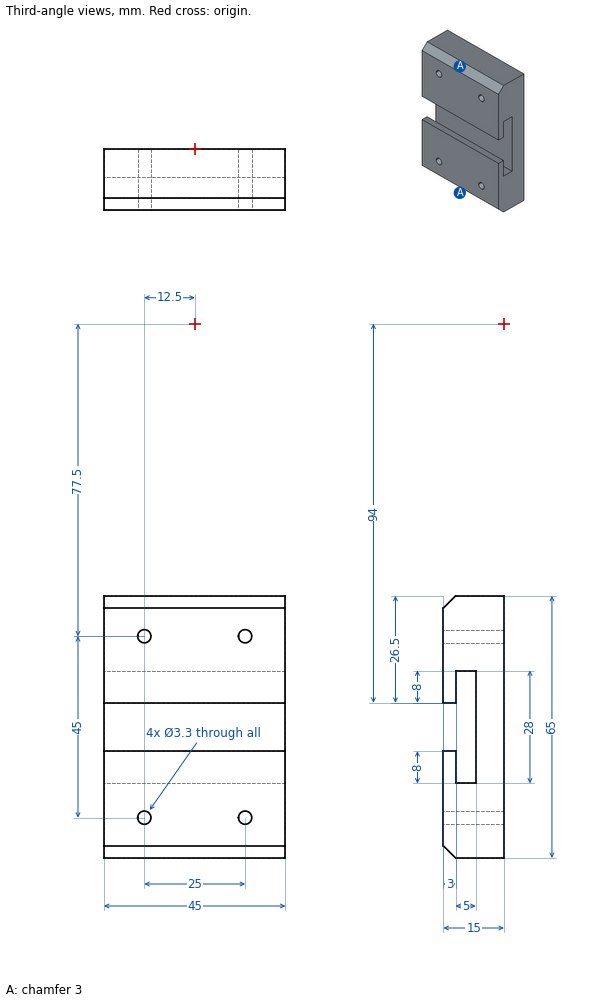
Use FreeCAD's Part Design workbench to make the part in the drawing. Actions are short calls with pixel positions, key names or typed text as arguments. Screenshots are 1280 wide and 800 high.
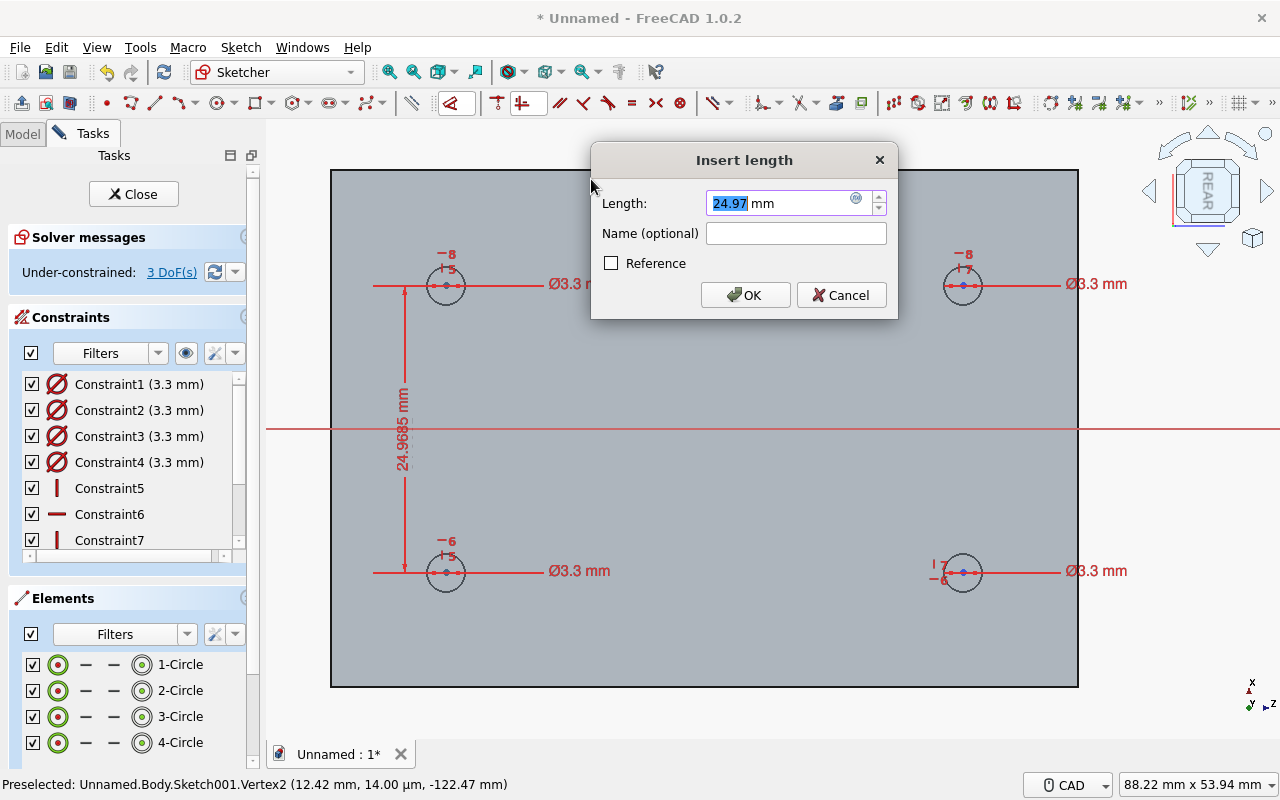
text(25)
key(Return)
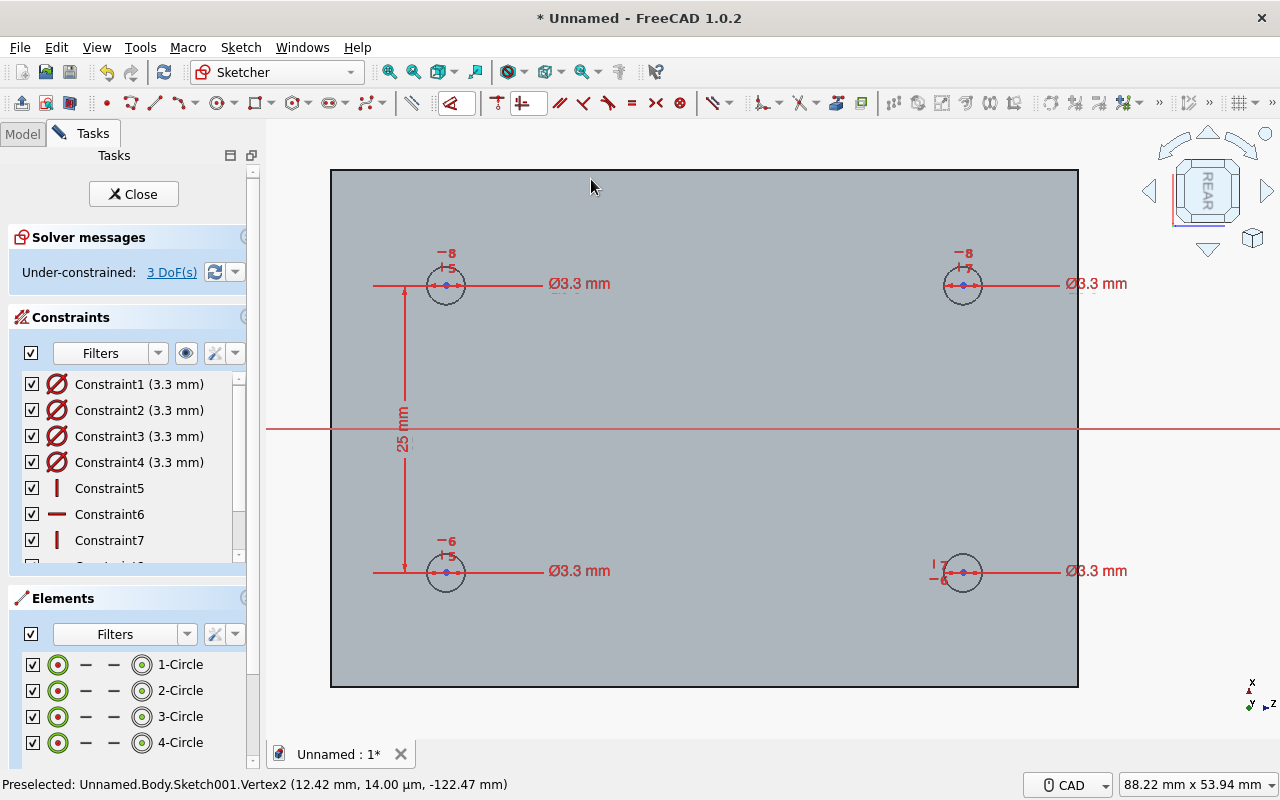
click(446, 573)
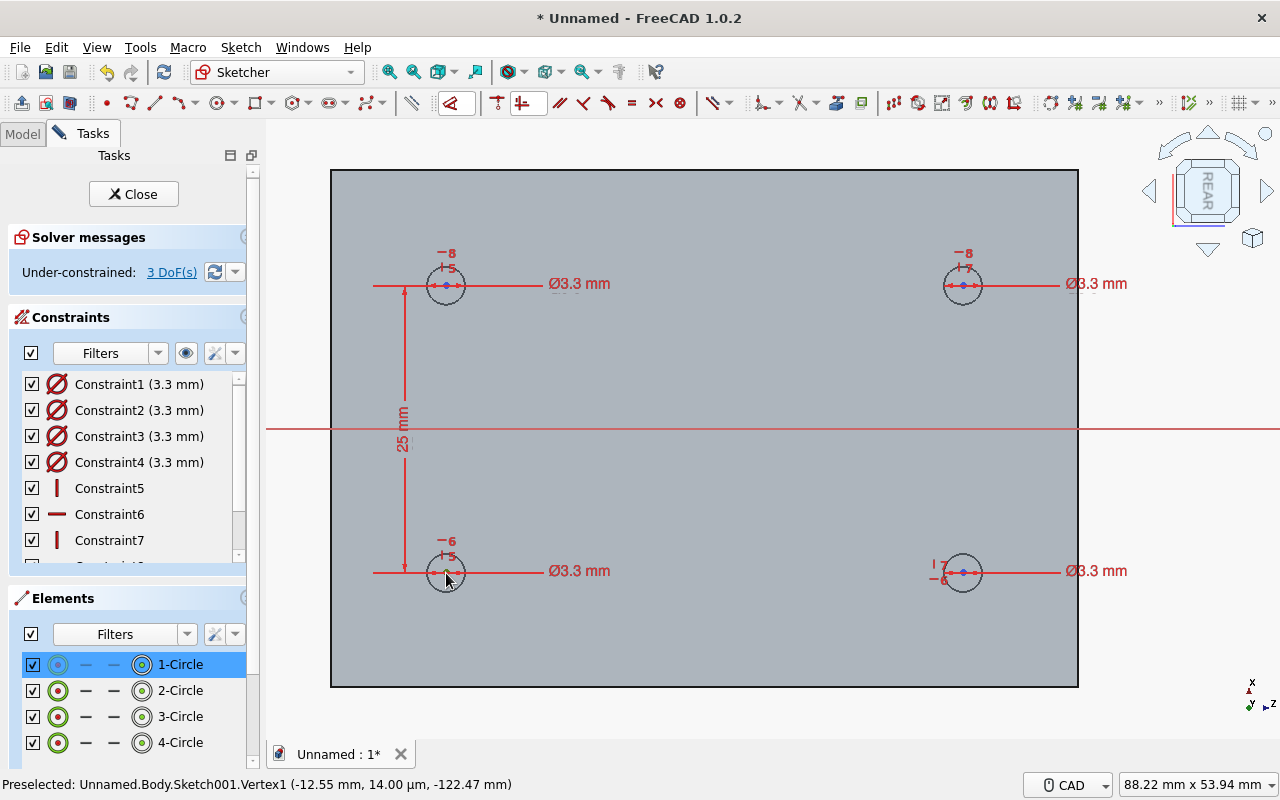
click(963, 573)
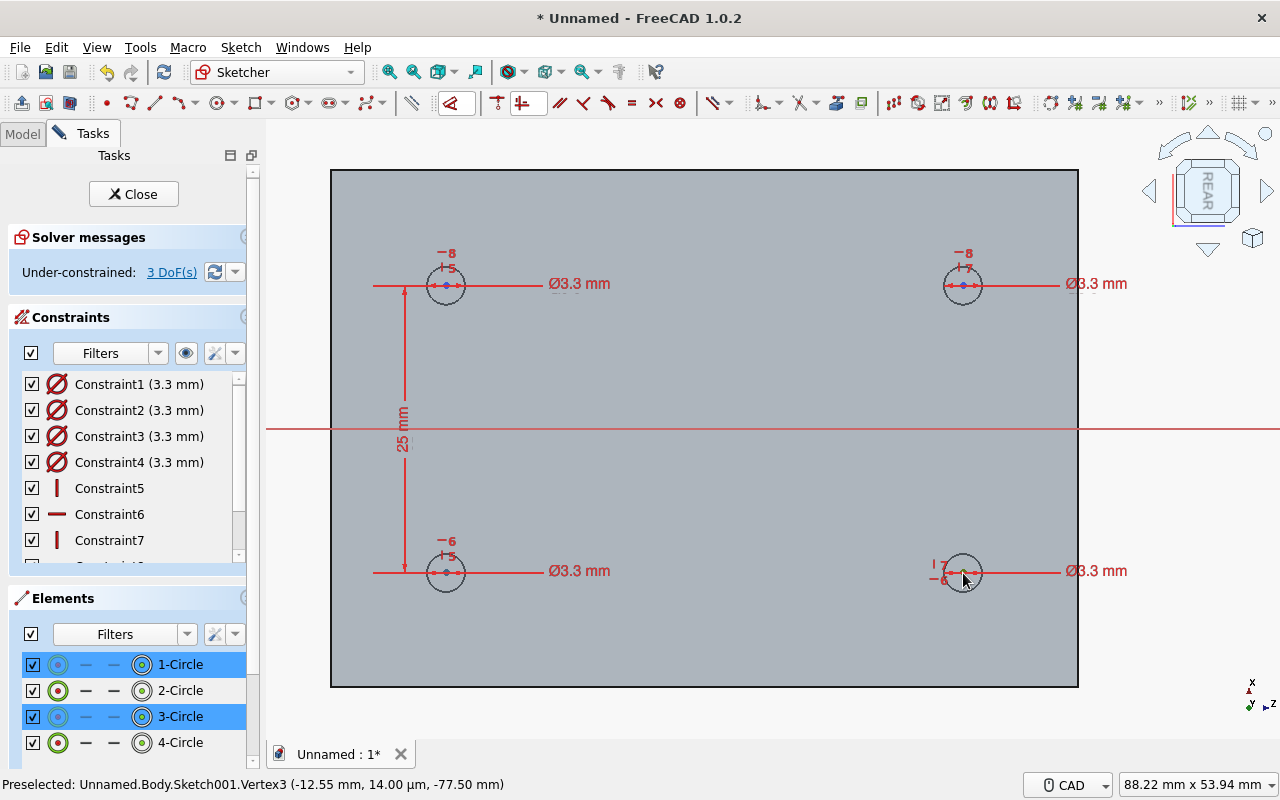
key(l)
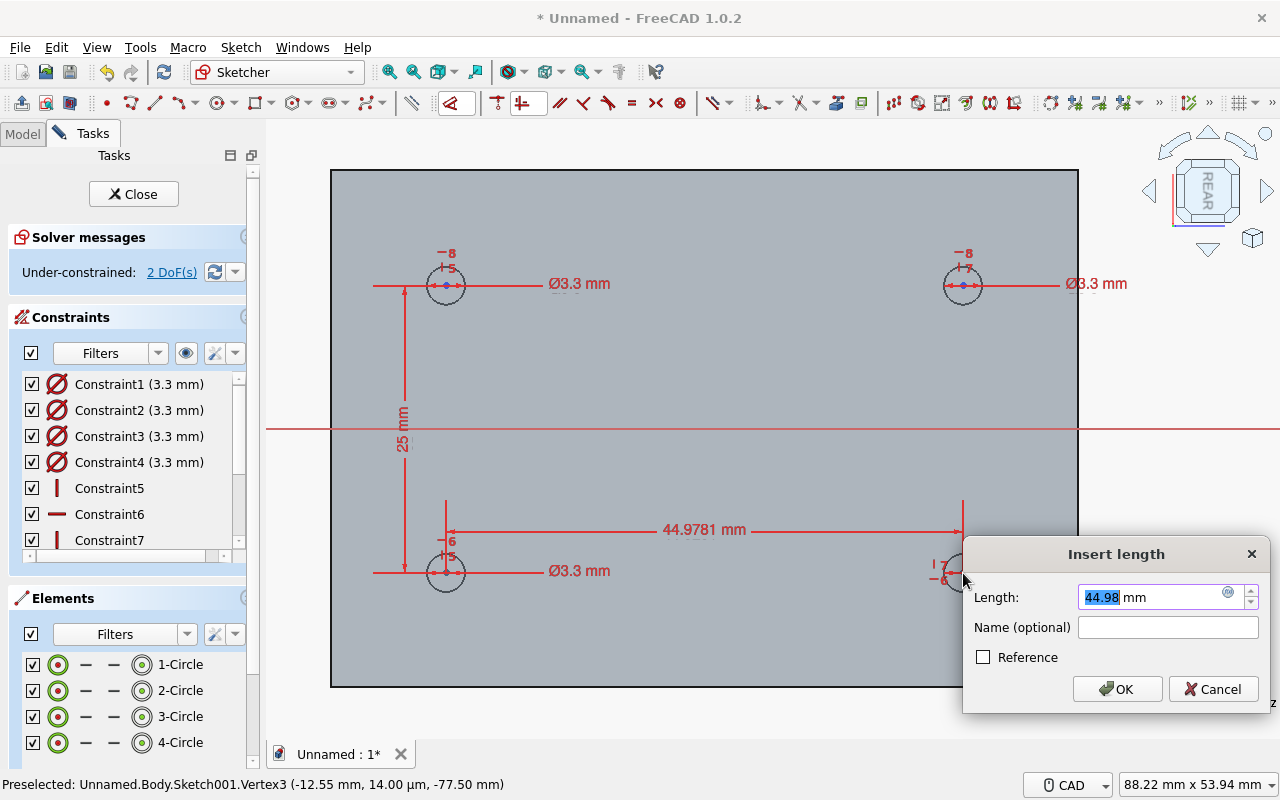
text(45)
key(Return)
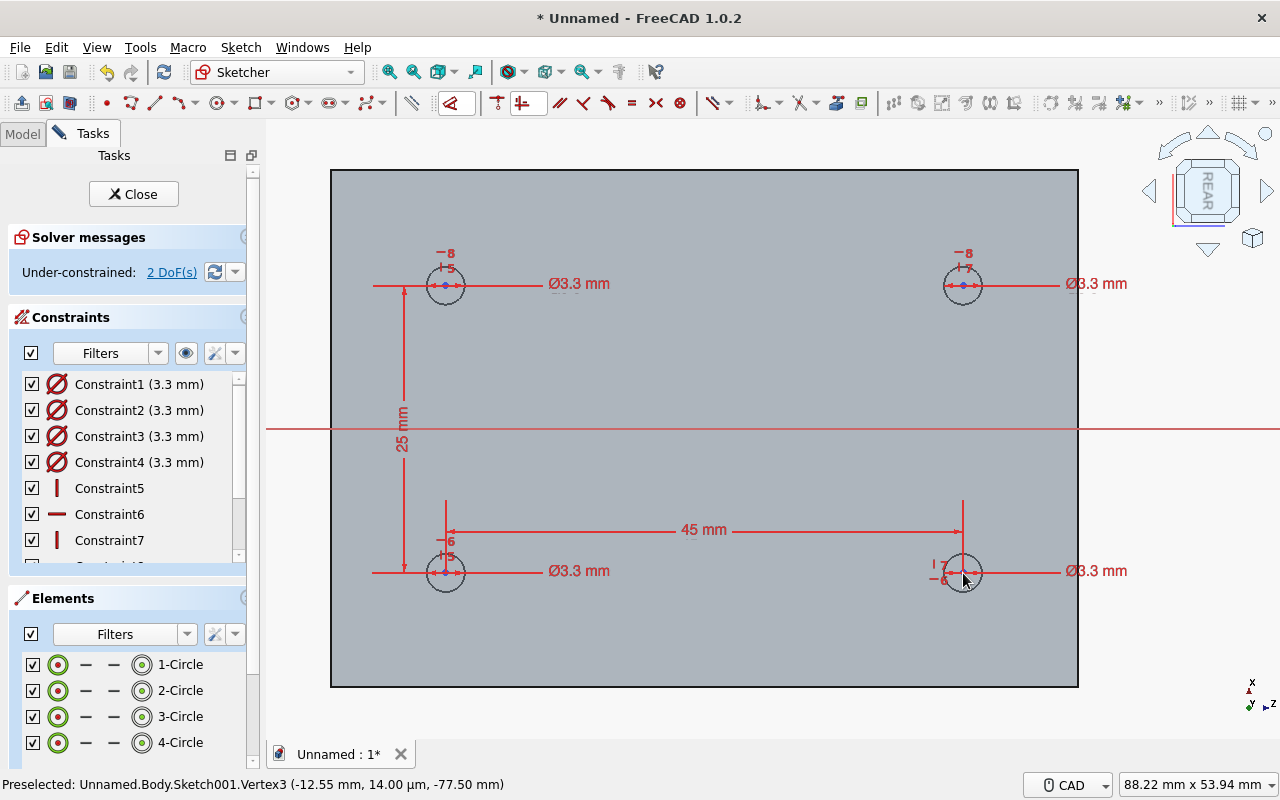
click(446, 573)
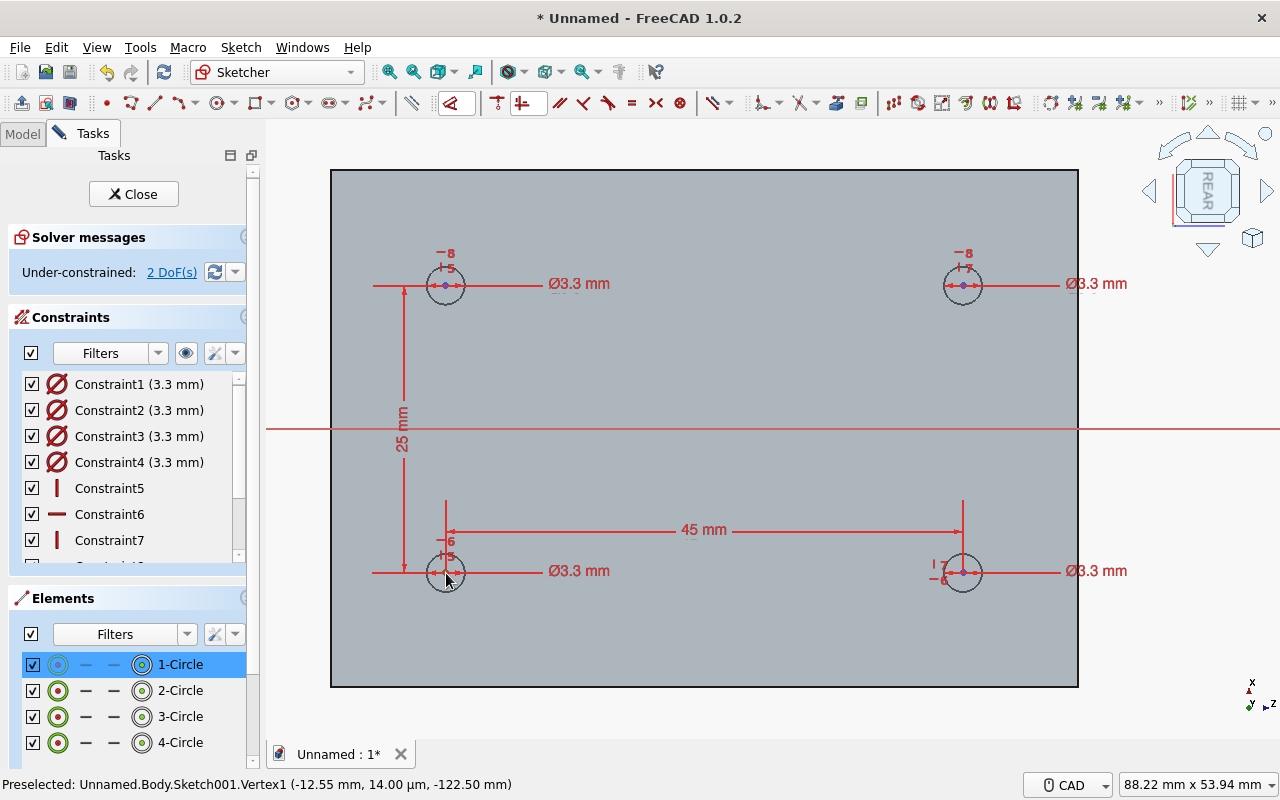
key(i)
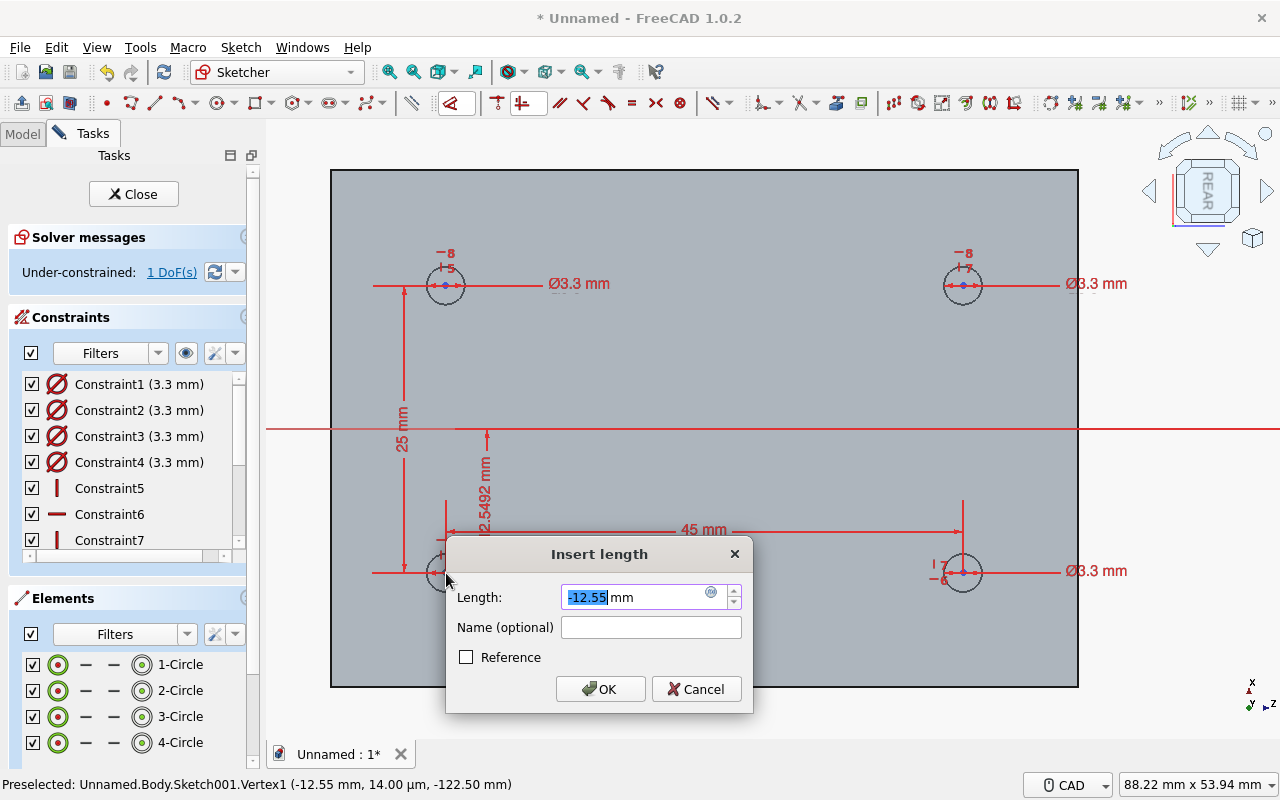
text(-12.5)
key(Return)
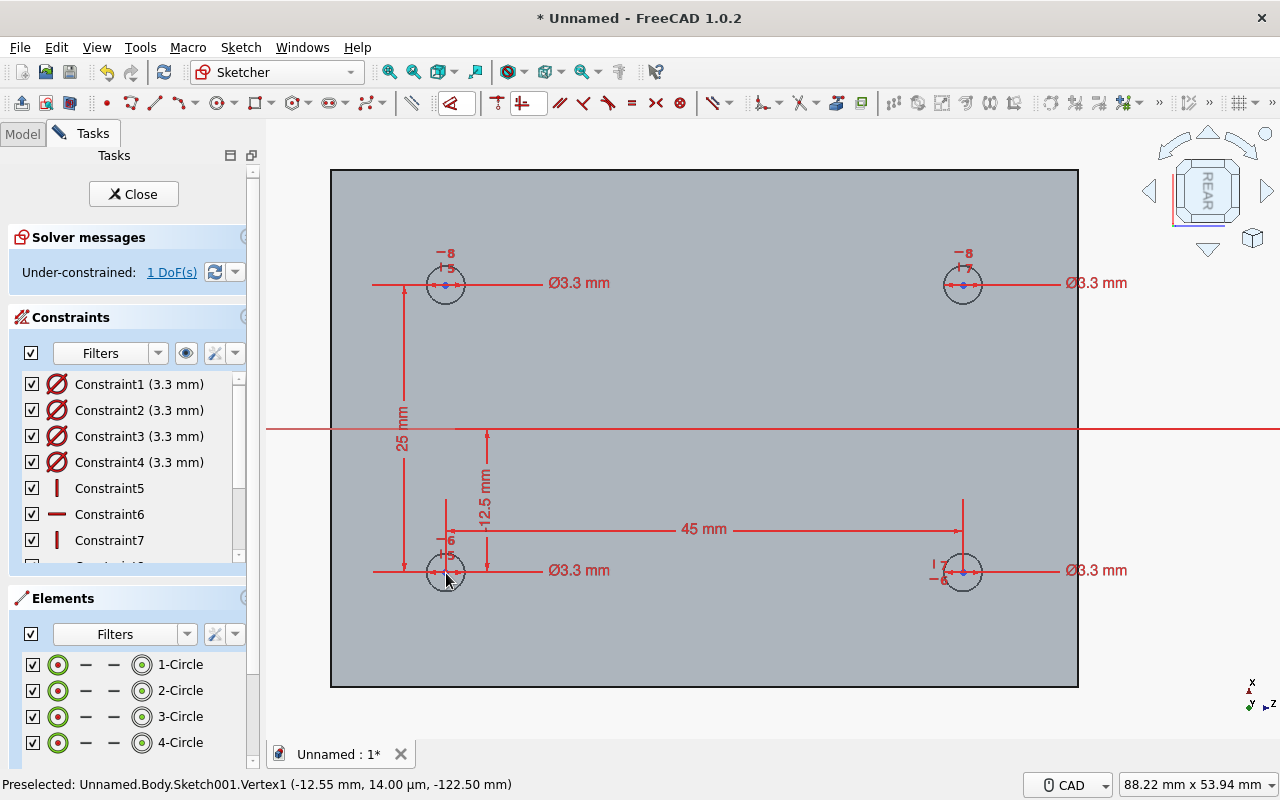
click(963, 572)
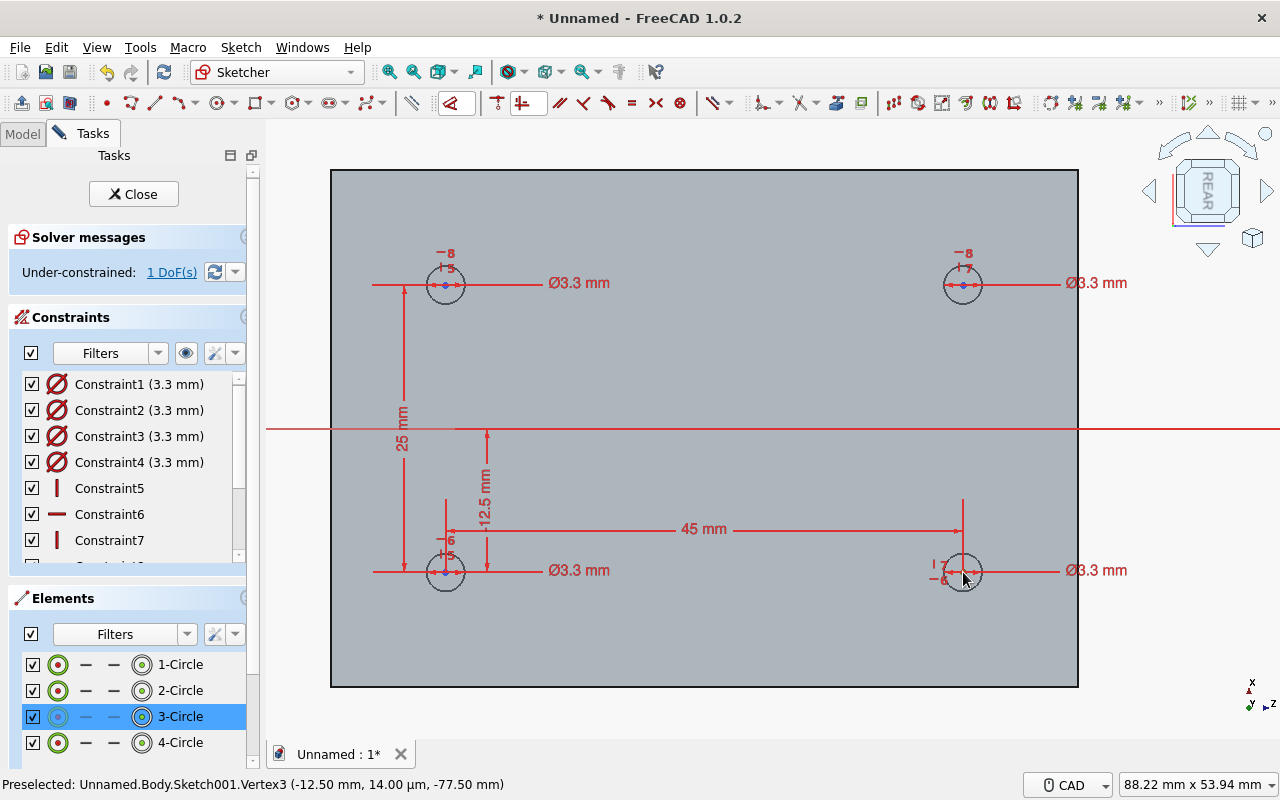
key(l)